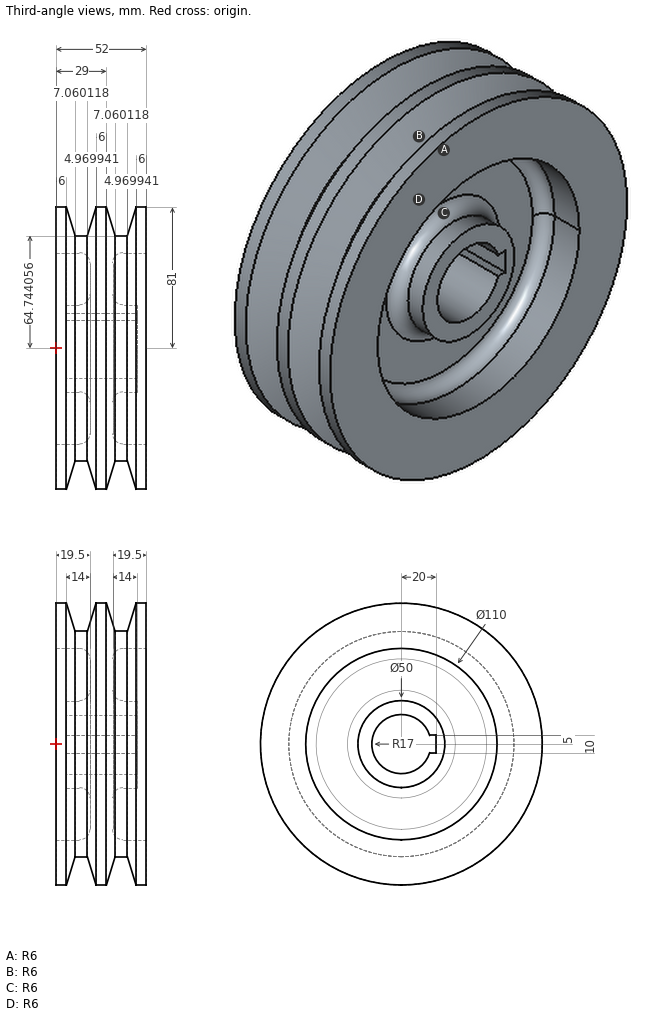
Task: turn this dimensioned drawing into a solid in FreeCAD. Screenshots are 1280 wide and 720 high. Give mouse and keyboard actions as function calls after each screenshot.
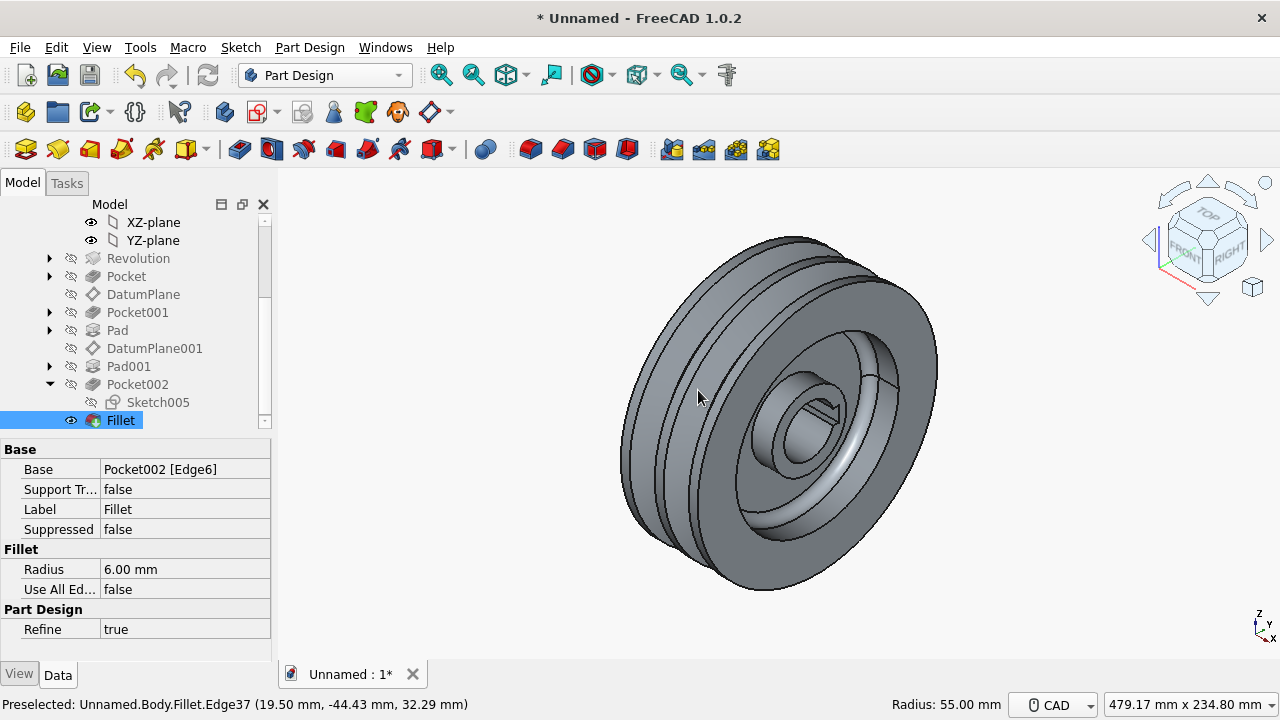
click(532, 150)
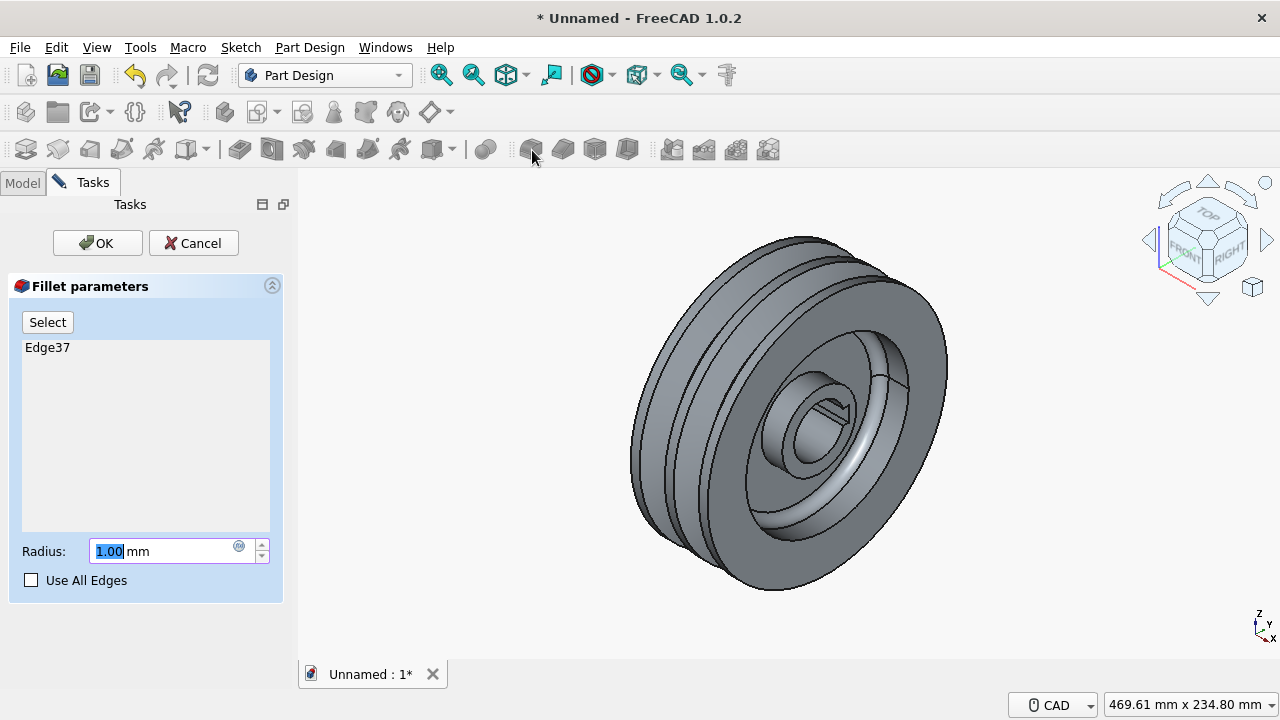
text(6)
key(Tab)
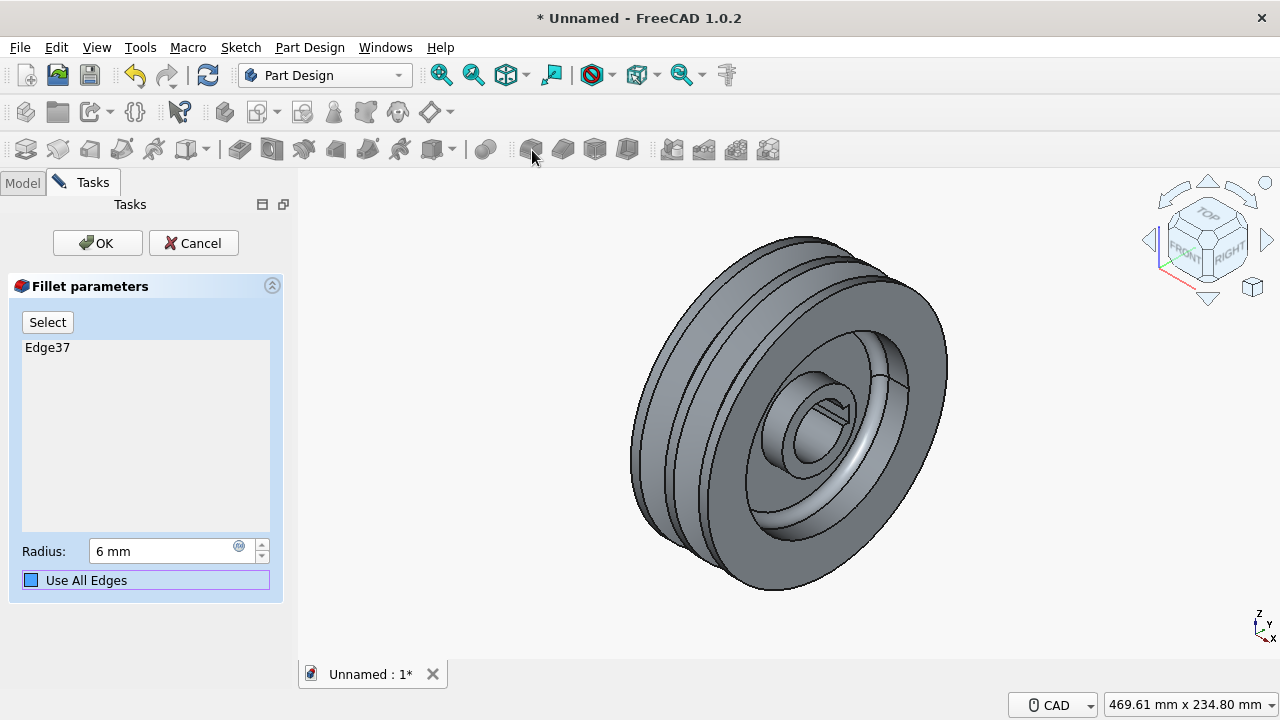
click(98, 243)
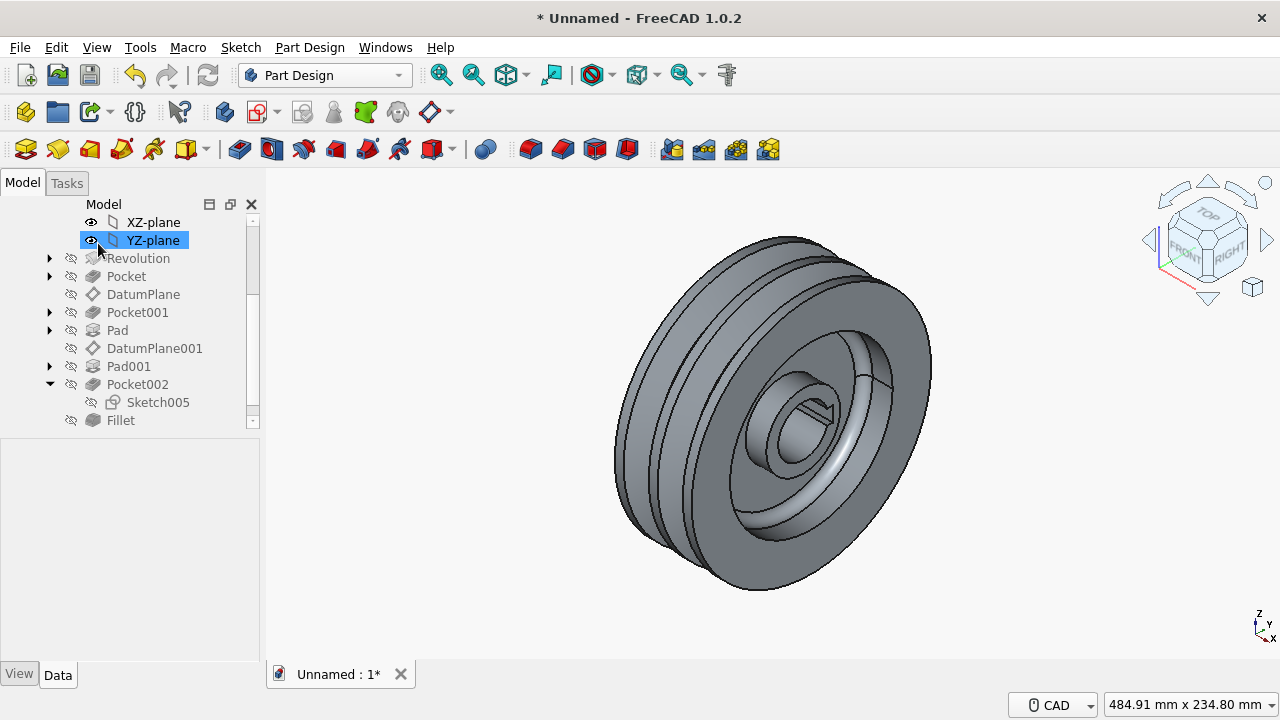
key(2)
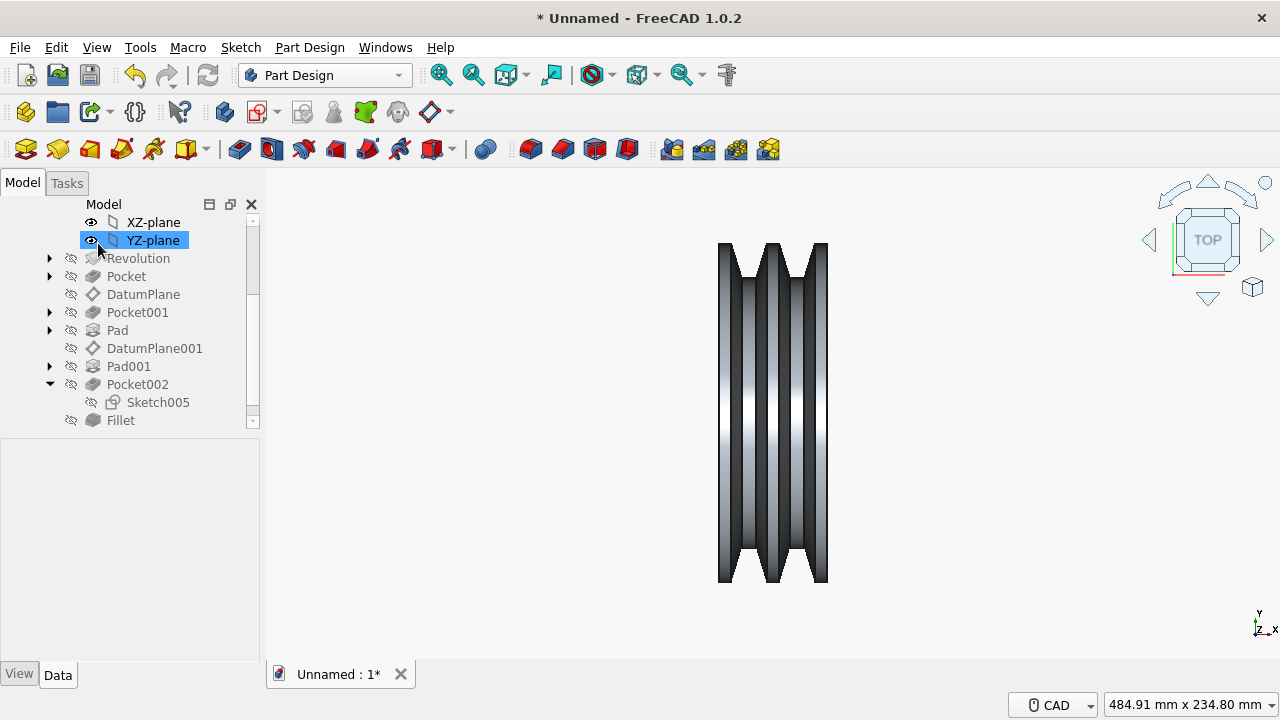
key(0)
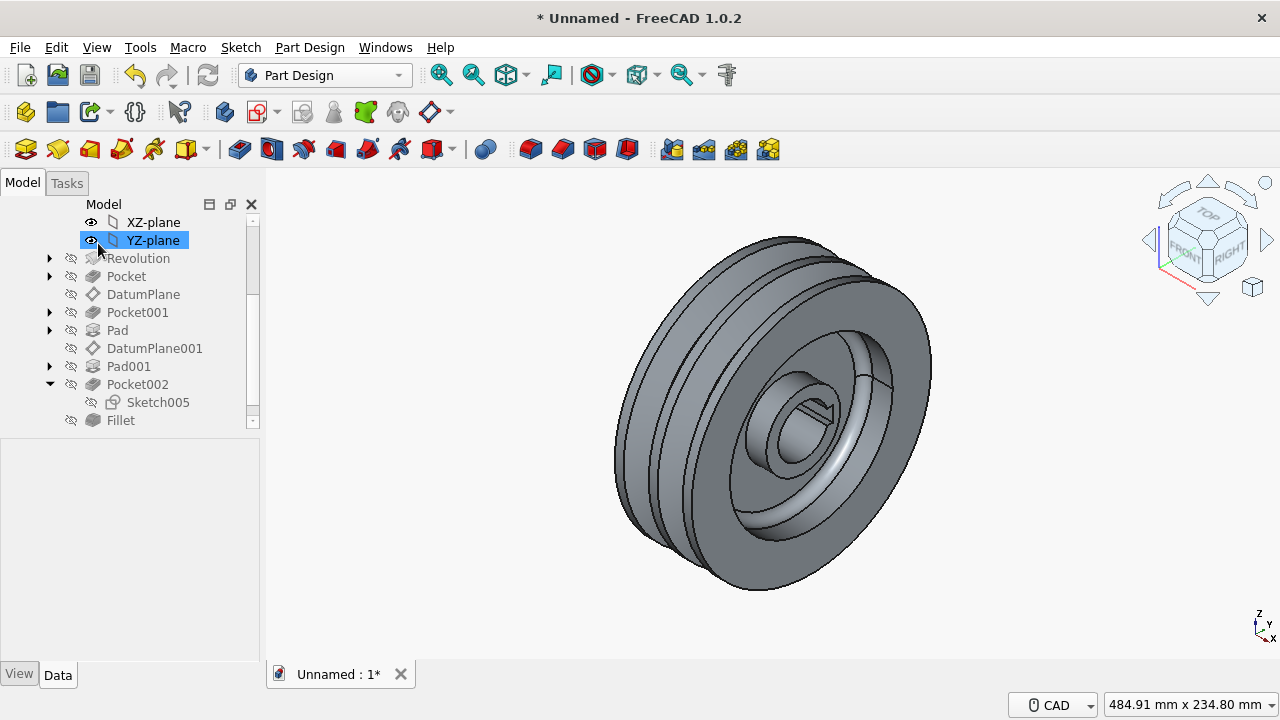
key(1)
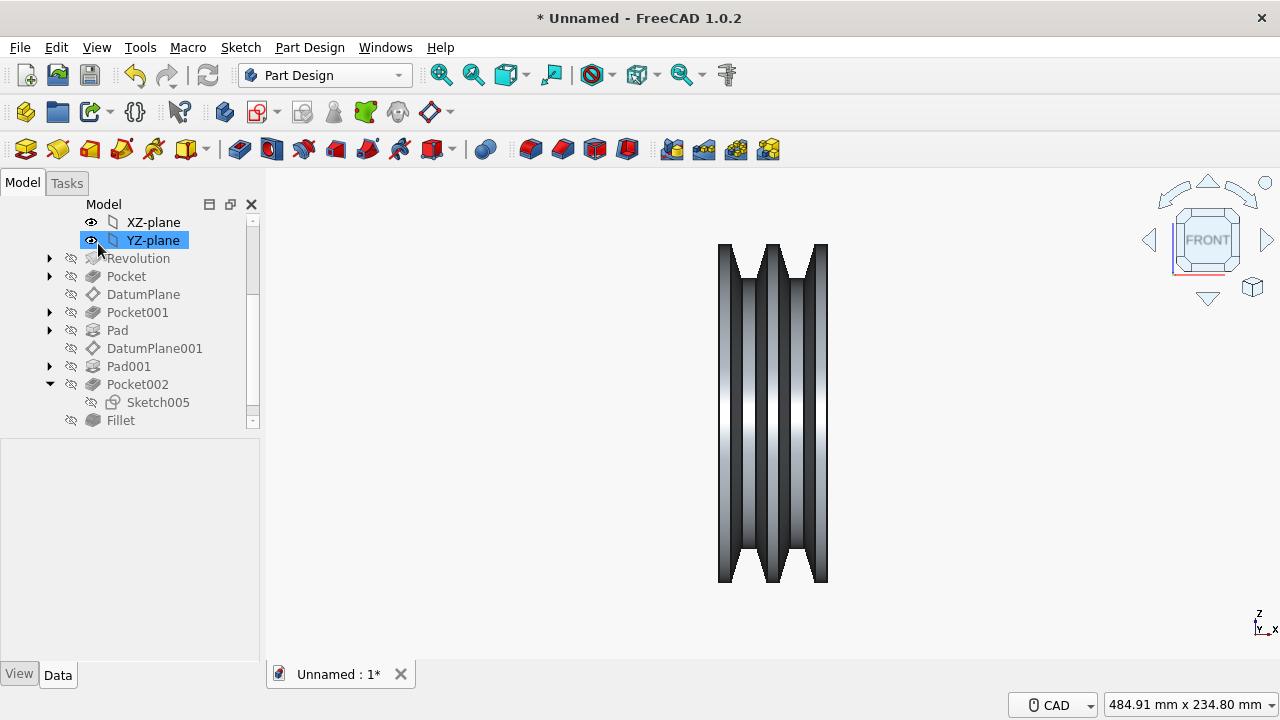
key(3)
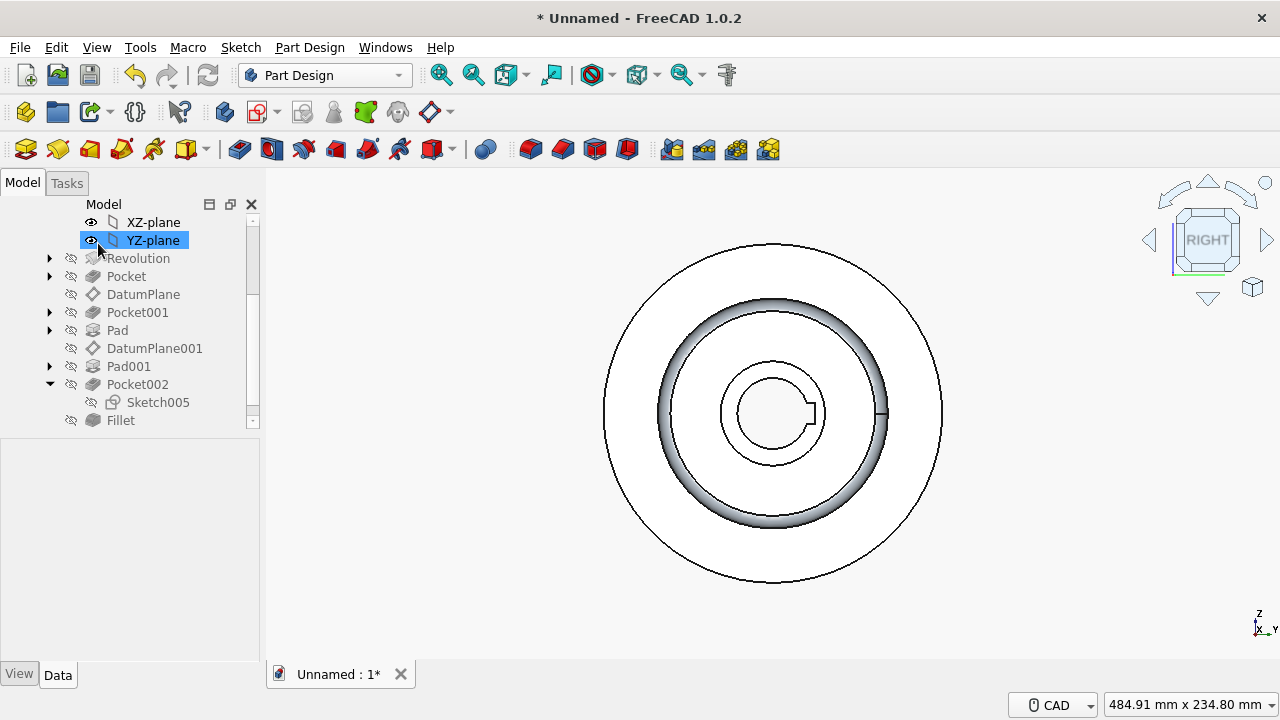
key(5)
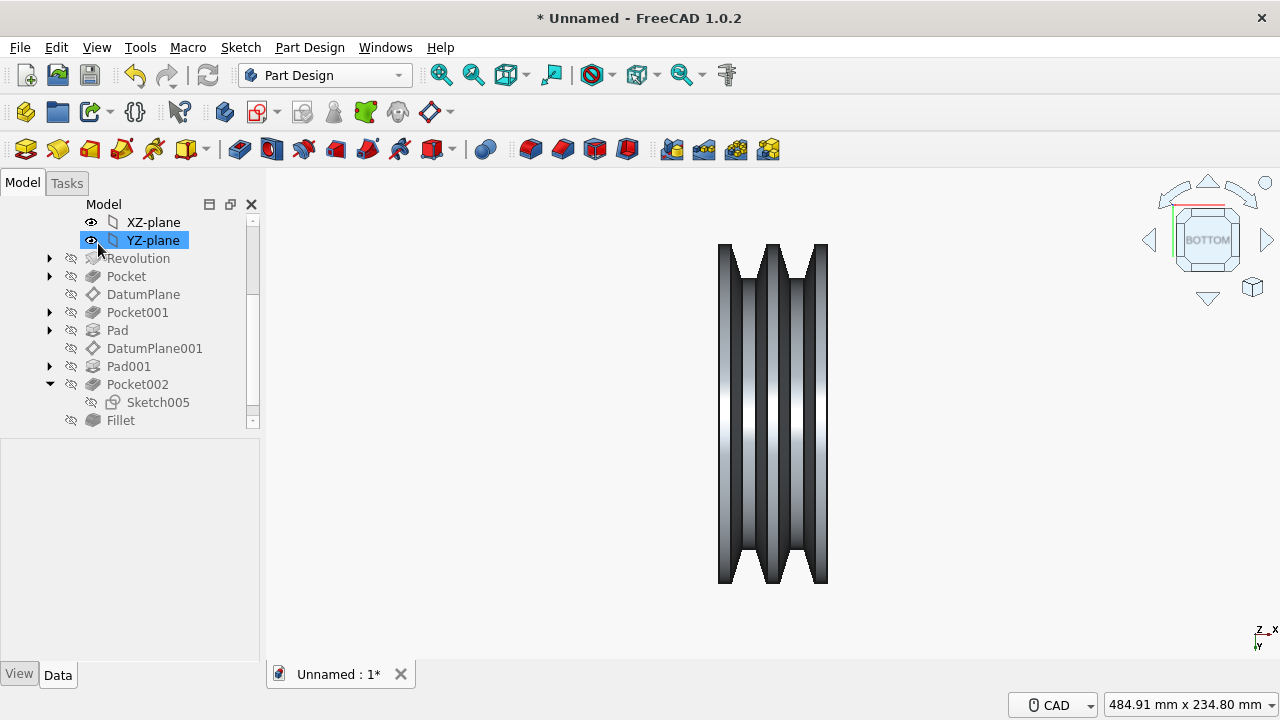
key(4)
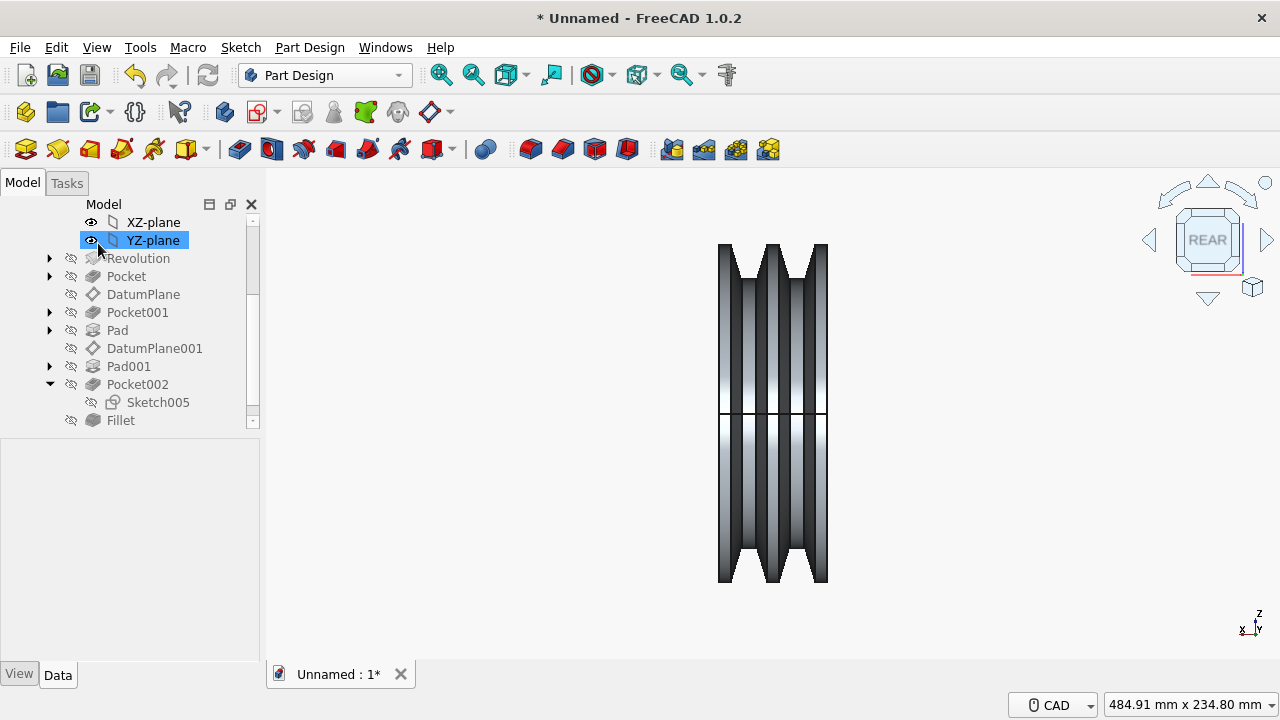
key(6)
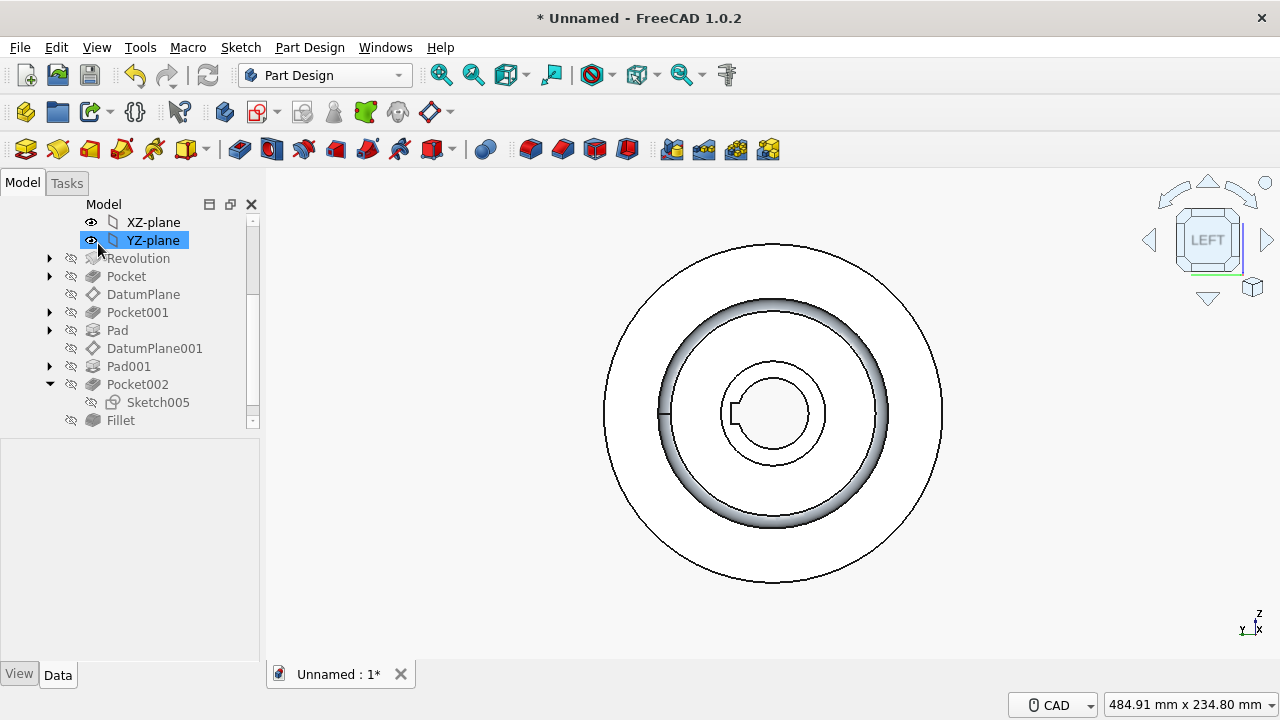
key(v)
key(3)